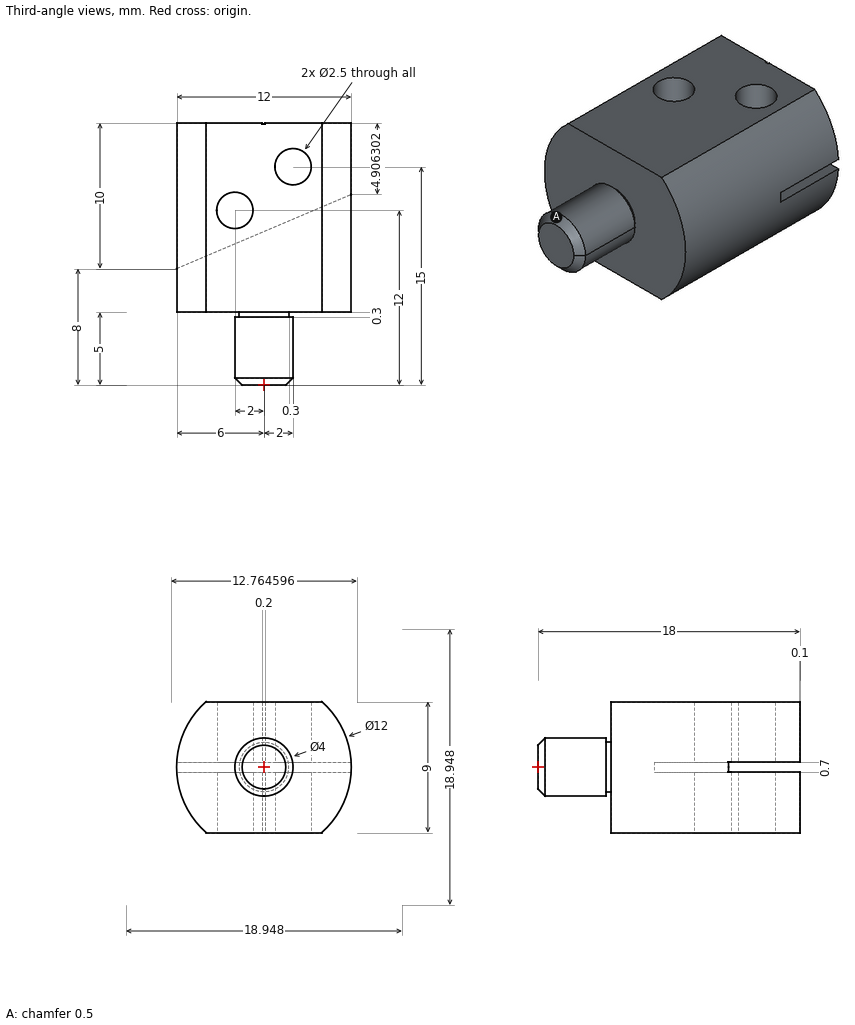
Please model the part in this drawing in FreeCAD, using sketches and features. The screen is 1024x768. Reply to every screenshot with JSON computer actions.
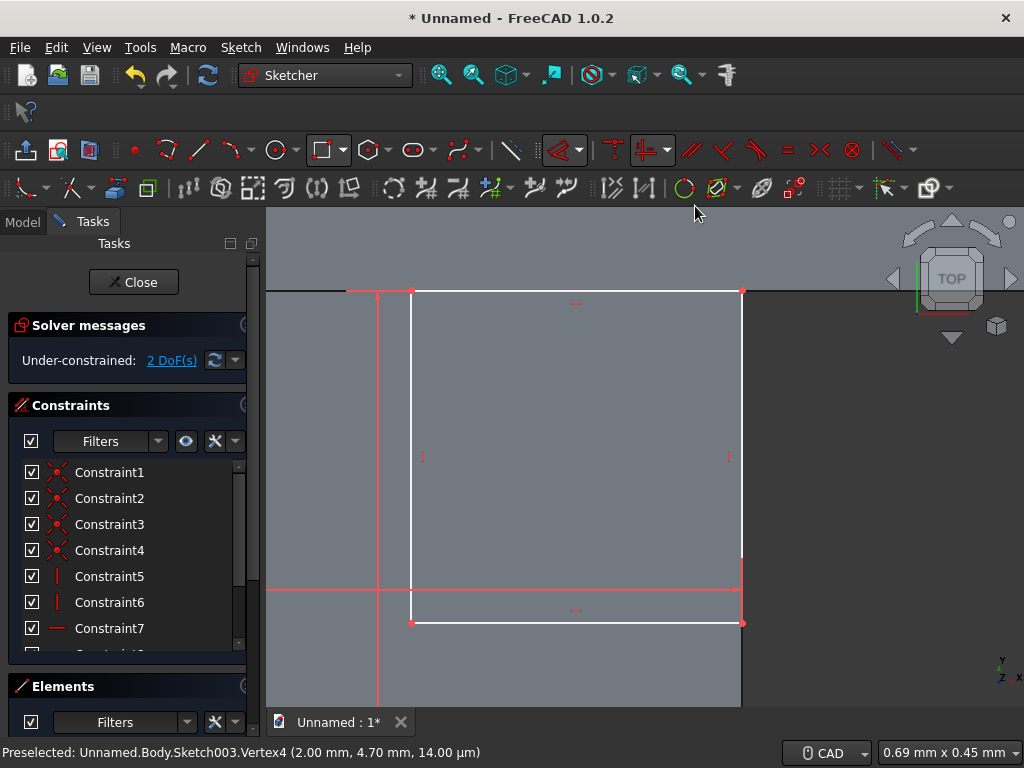
{"action": "left_click", "coordinate": [411, 391]}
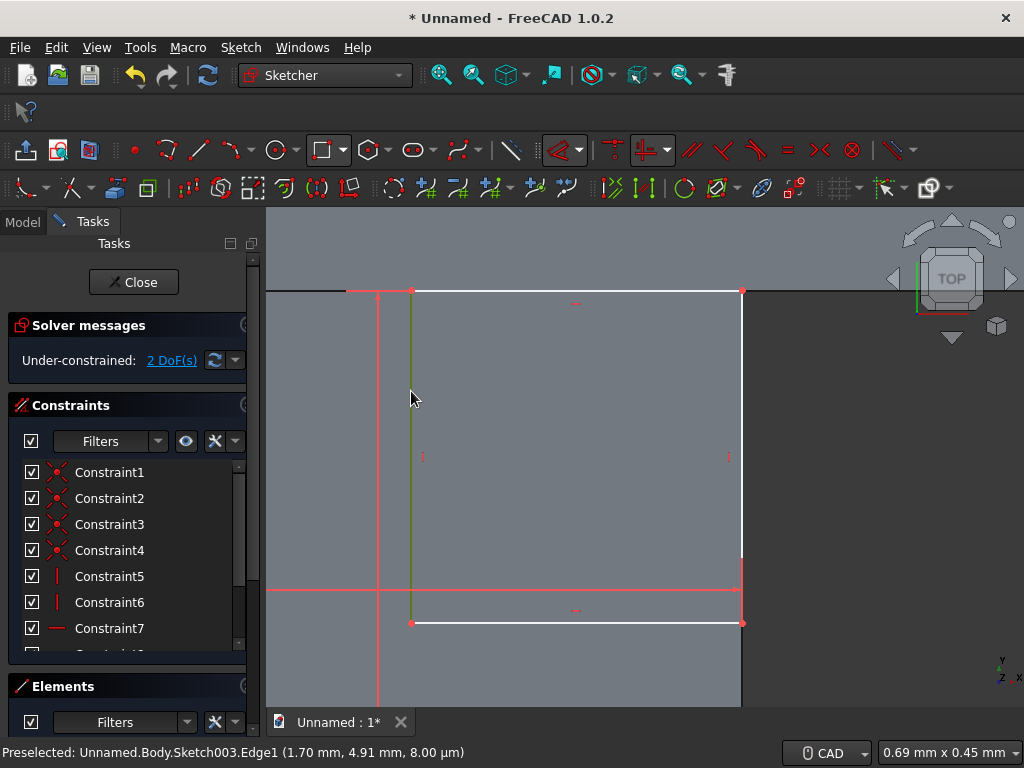
{"action": "key", "text": "i"}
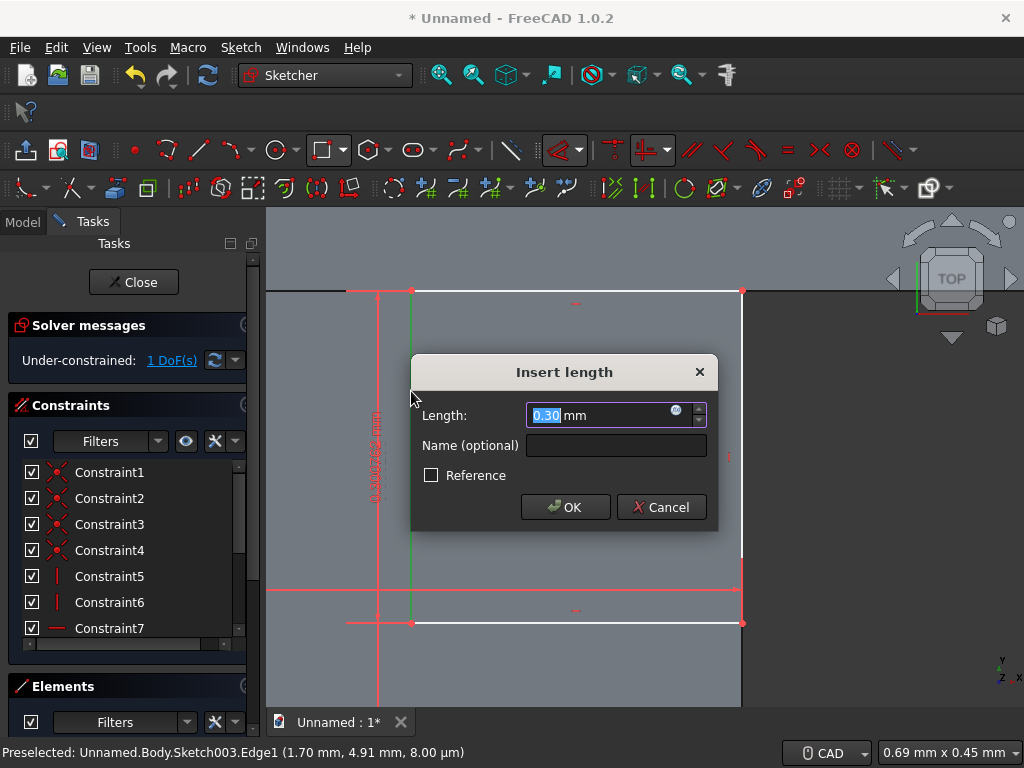
{"action": "type", "text": "0.3"}
{"action": "key", "text": "Return"}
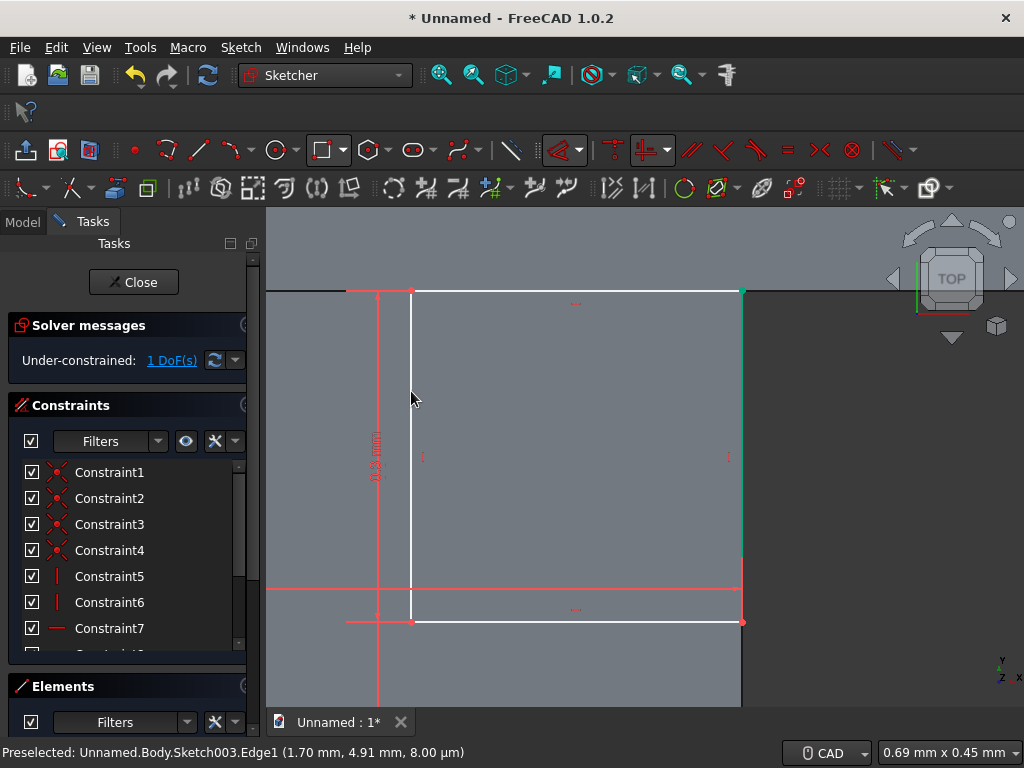
{"action": "left_click", "coordinate": [510, 622]}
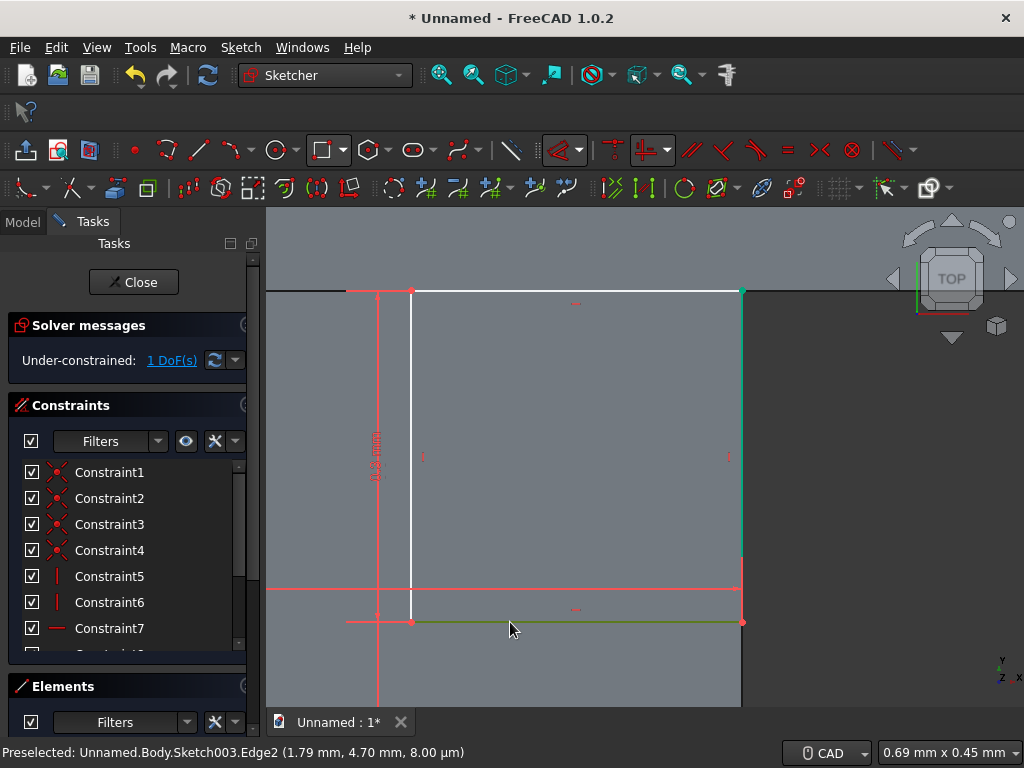
{"action": "left_click", "coordinate": [582, 150]}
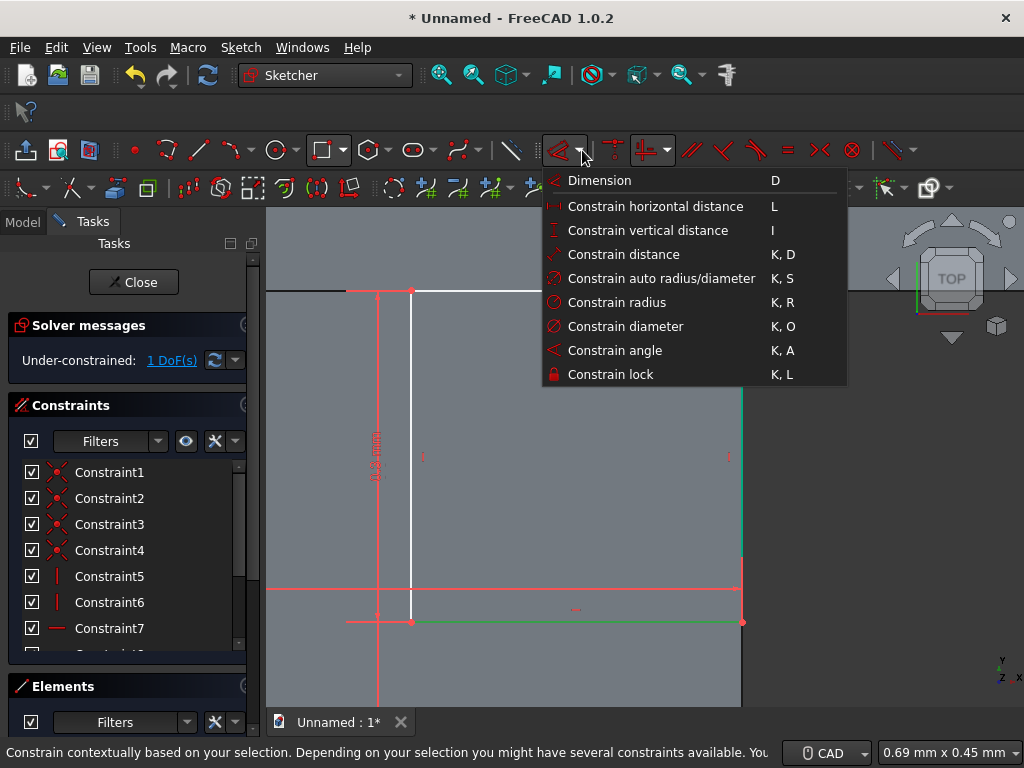
{"action": "left_click", "coordinate": [695, 206]}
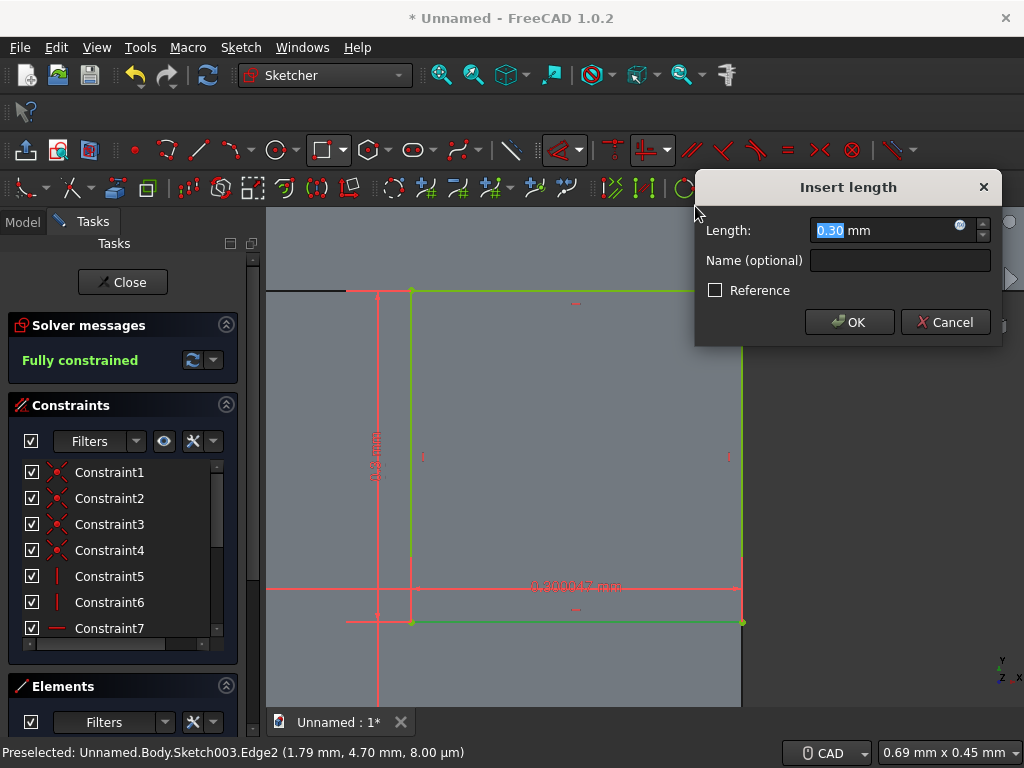
{"action": "type", "text": "0.3"}
{"action": "key", "text": "Return"}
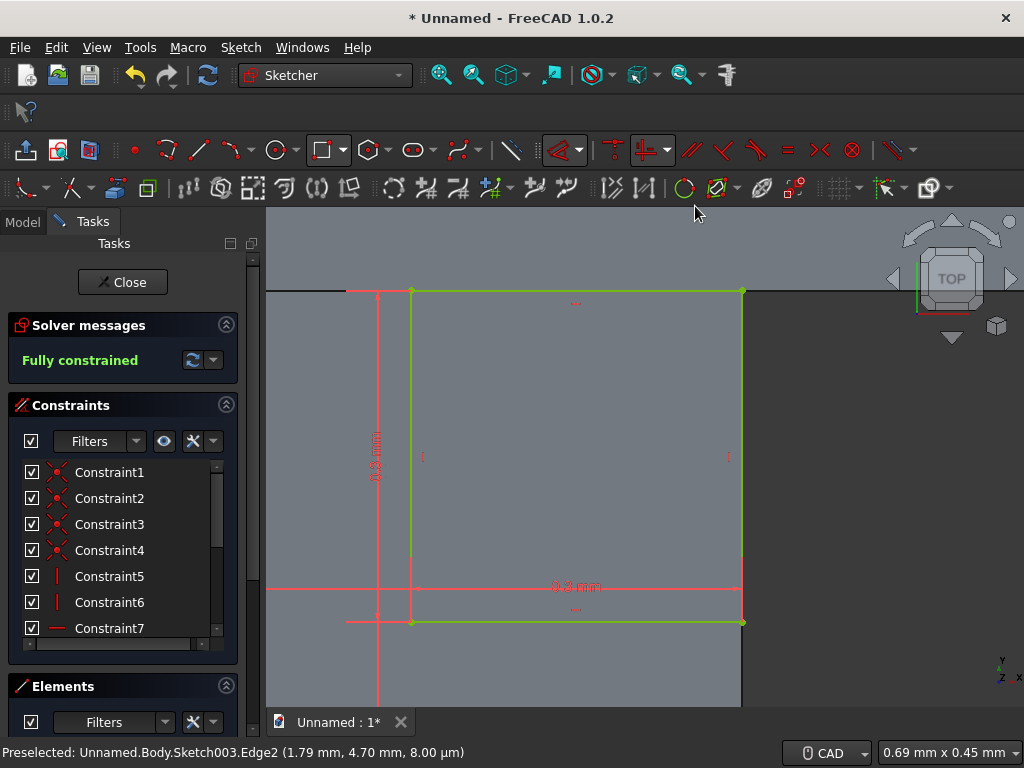
{"action": "left_click", "coordinate": [123, 282]}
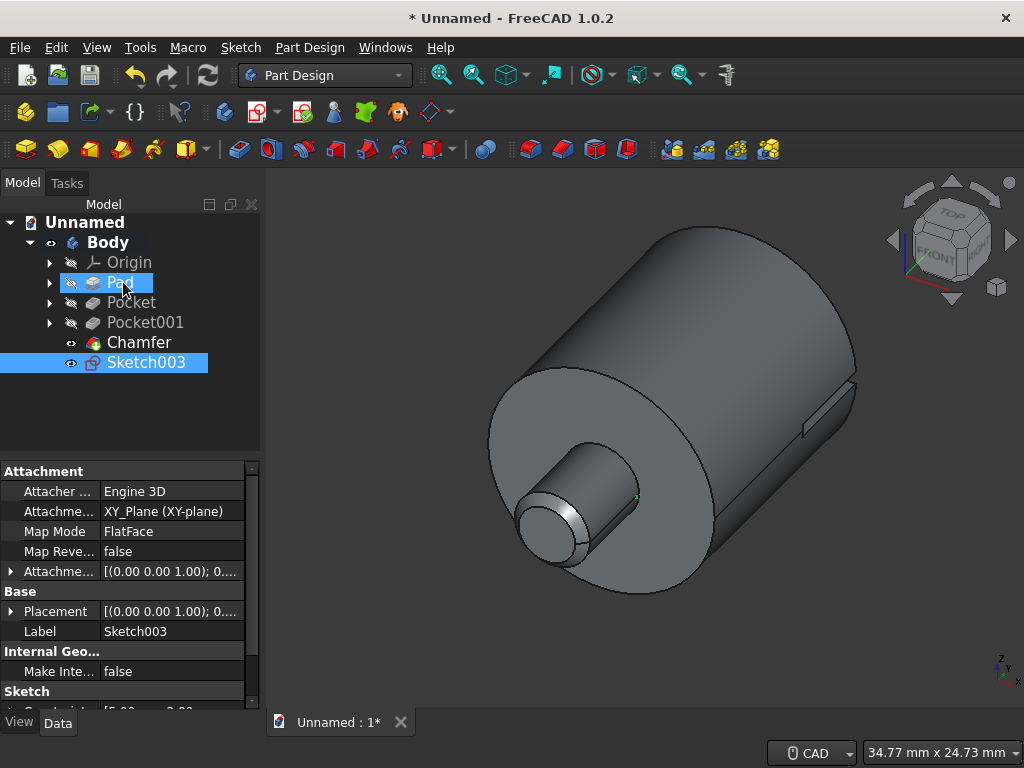
{"action": "left_click", "coordinate": [304, 150]}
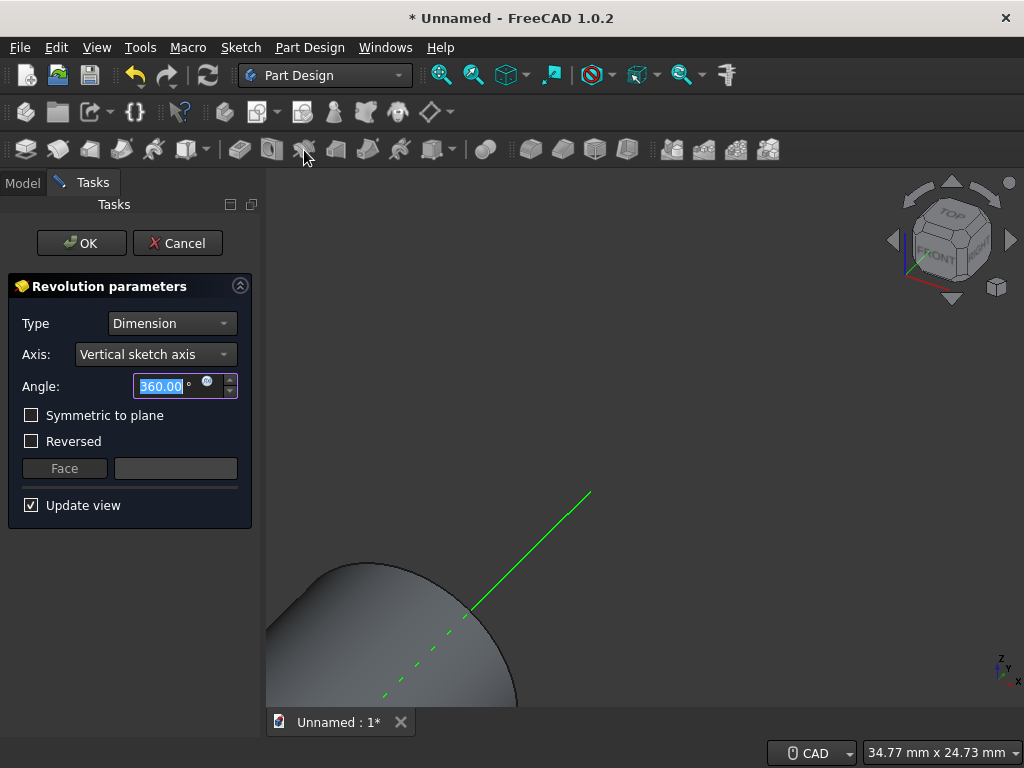
{"action": "left_click", "coordinate": [82, 243]}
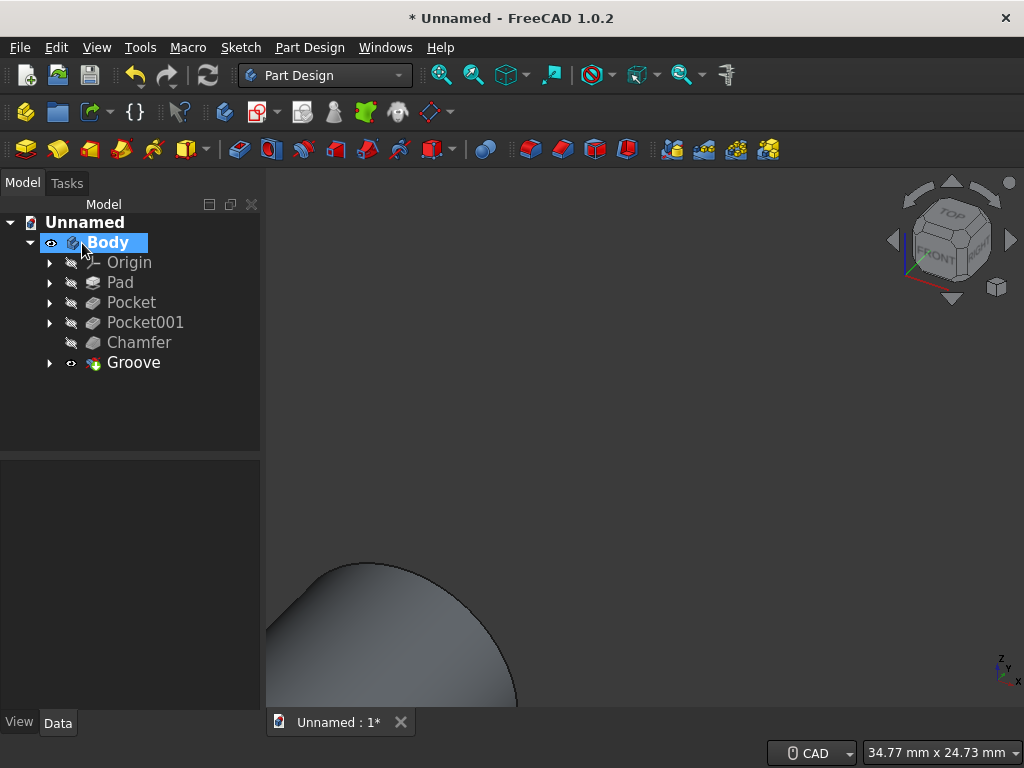
{"action": "left_click", "coordinate": [442, 76]}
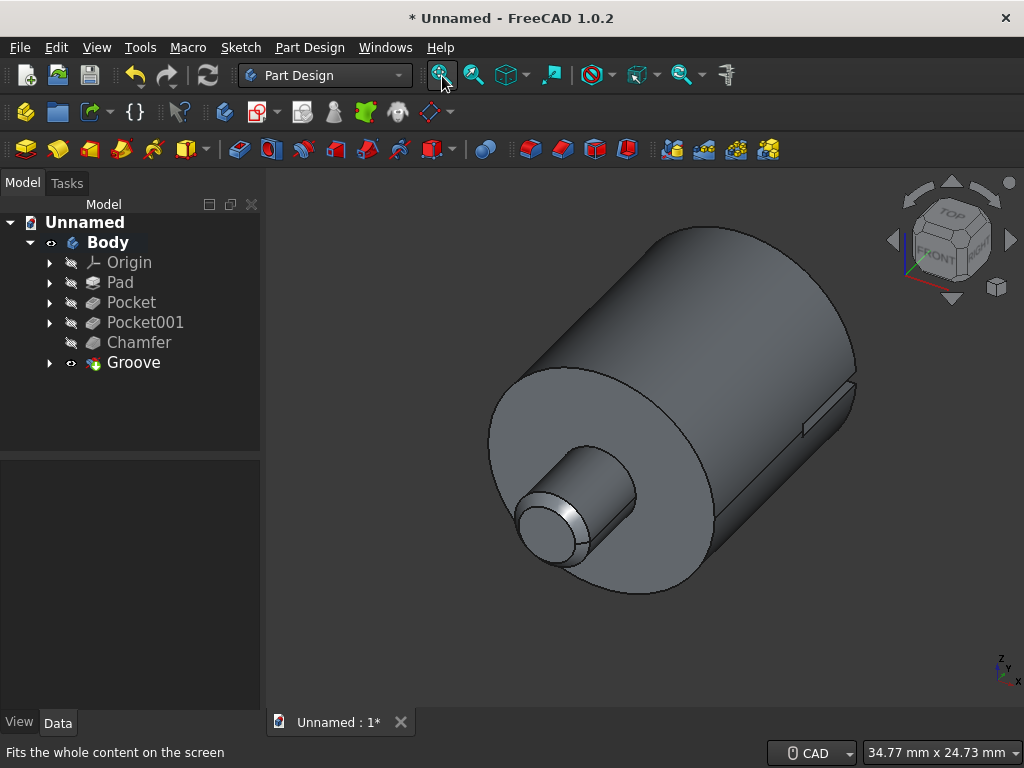
{"action": "key", "text": "4"}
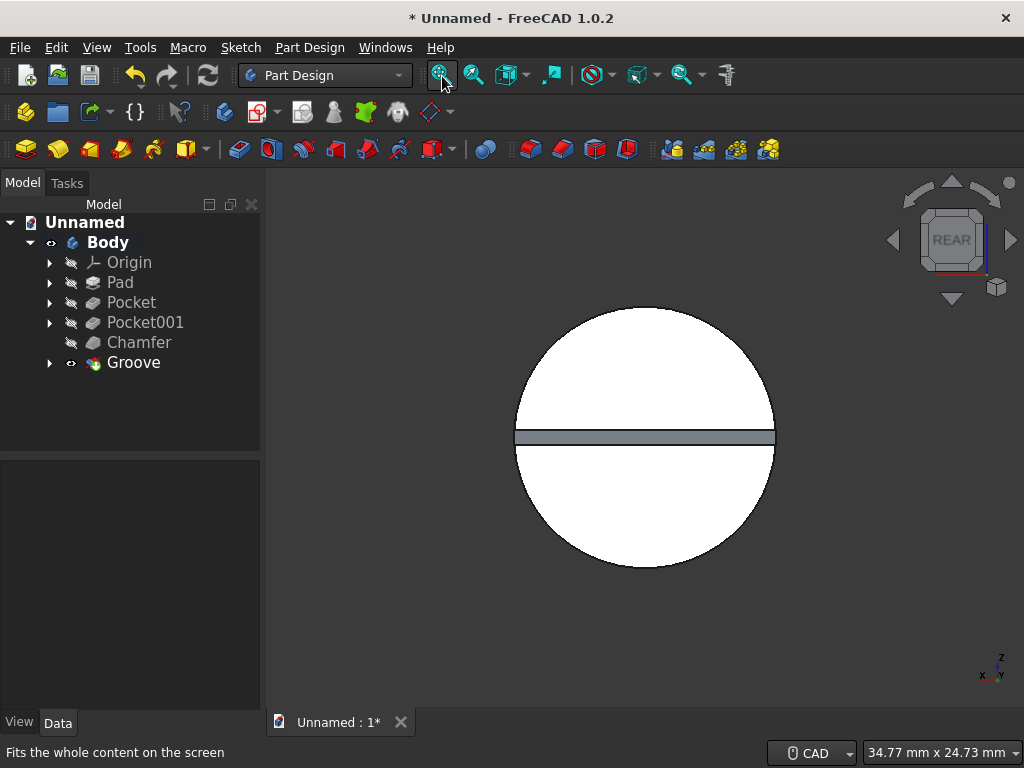
{"action": "left_click", "coordinate": [645, 506]}